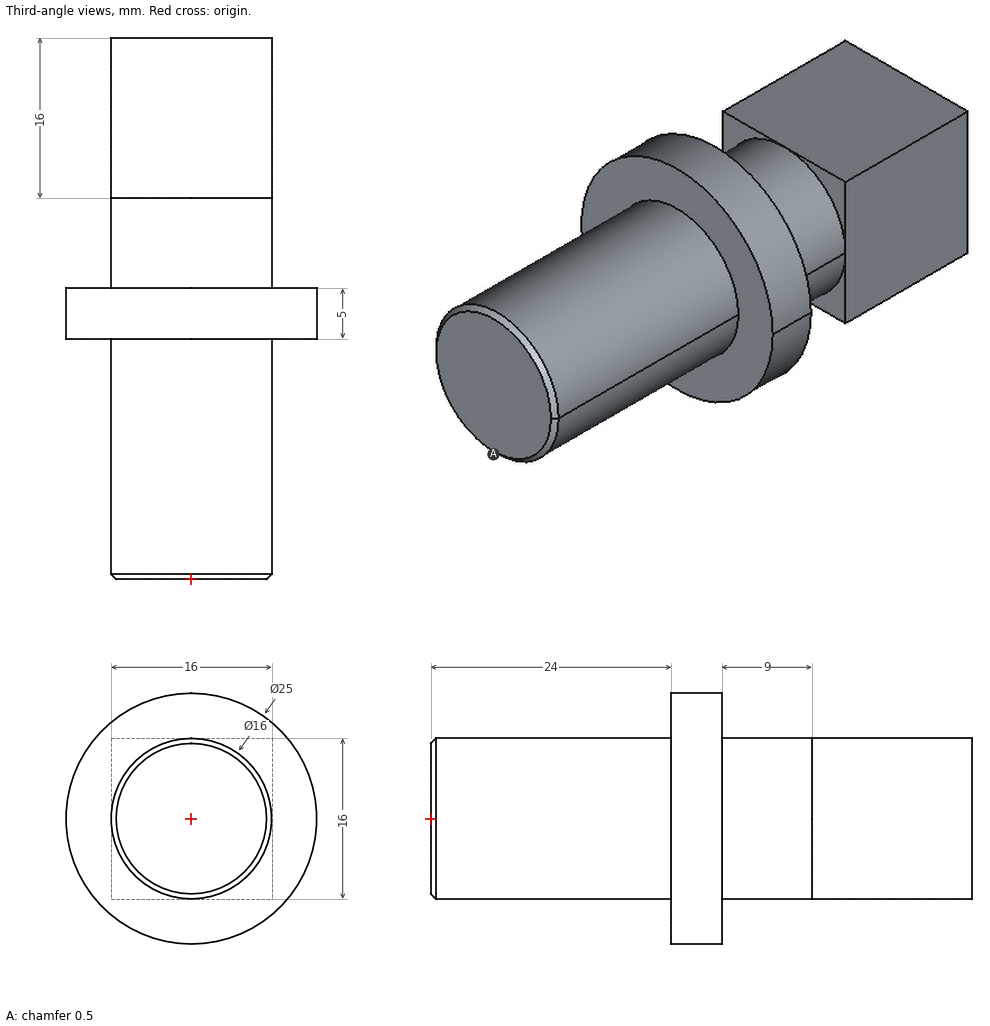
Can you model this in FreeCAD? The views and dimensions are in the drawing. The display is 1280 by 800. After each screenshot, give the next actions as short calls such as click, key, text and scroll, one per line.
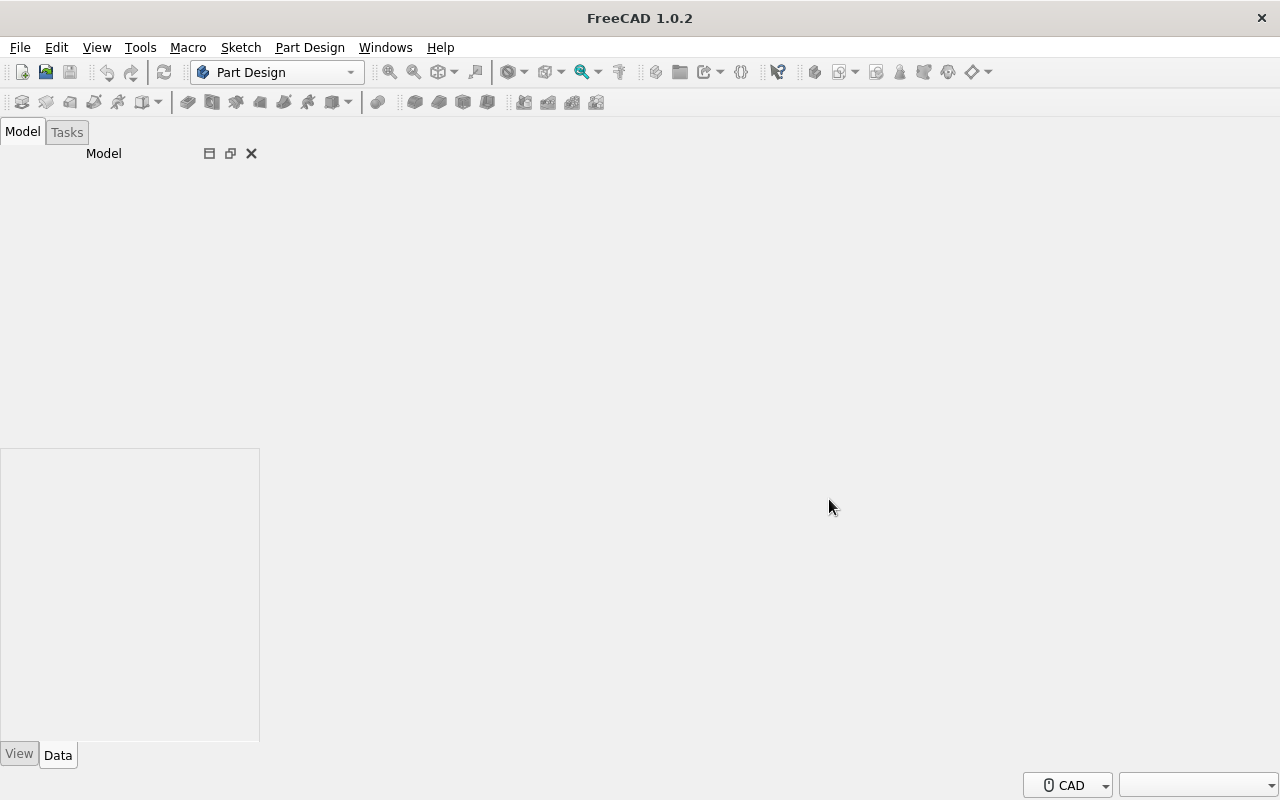
click(22, 72)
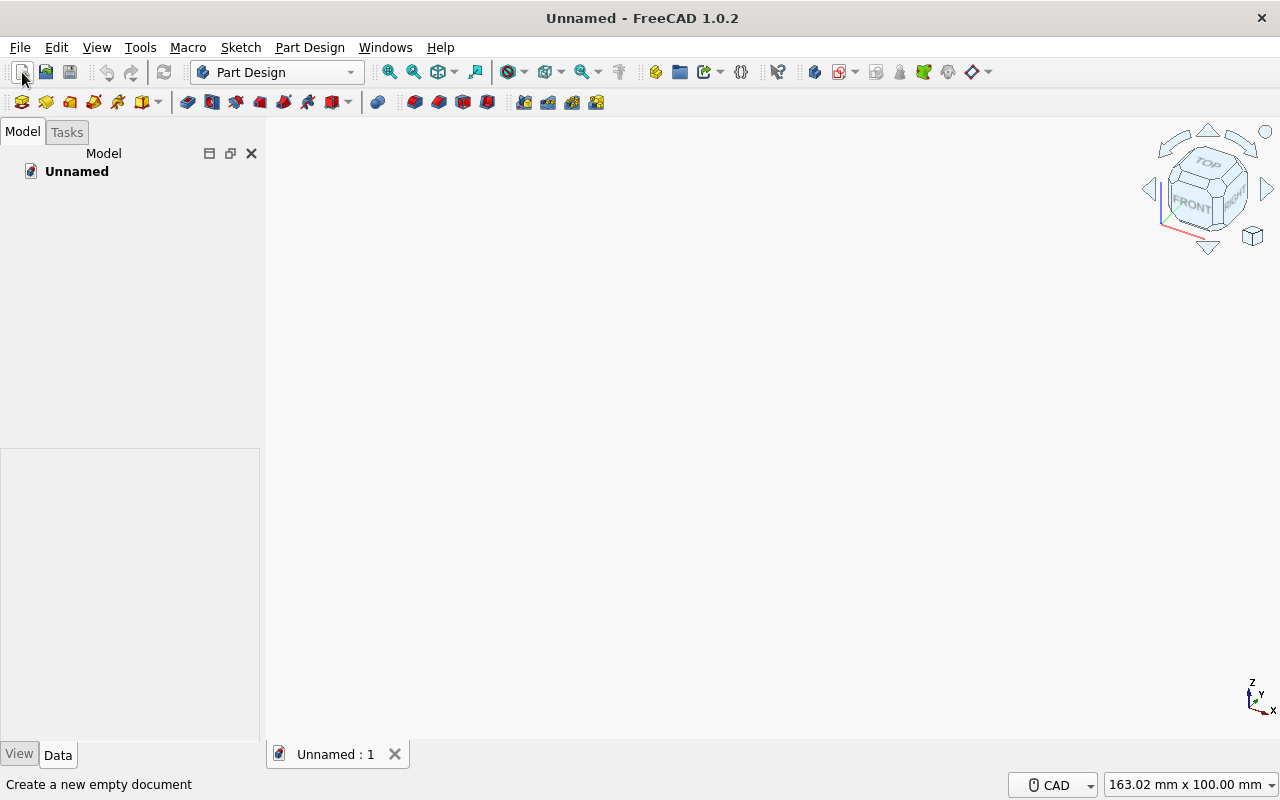
click(840, 72)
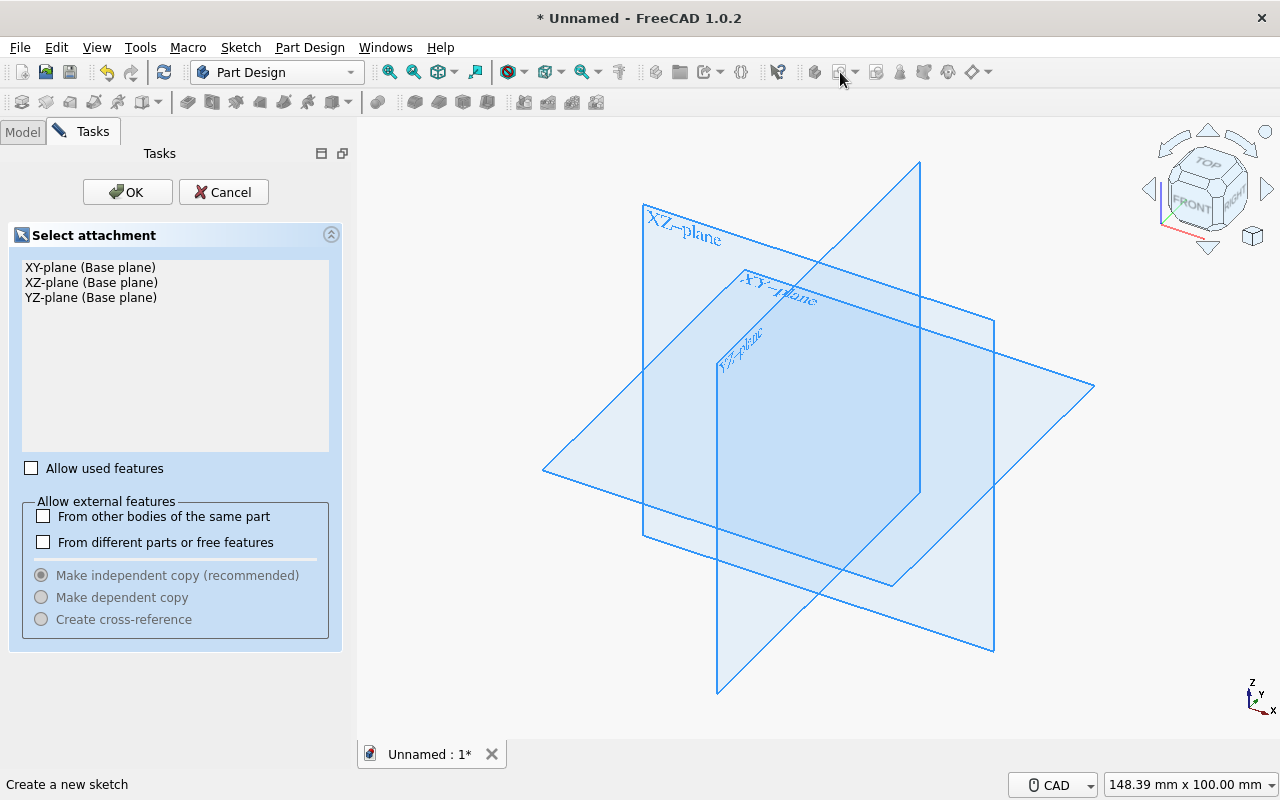
click(82, 282)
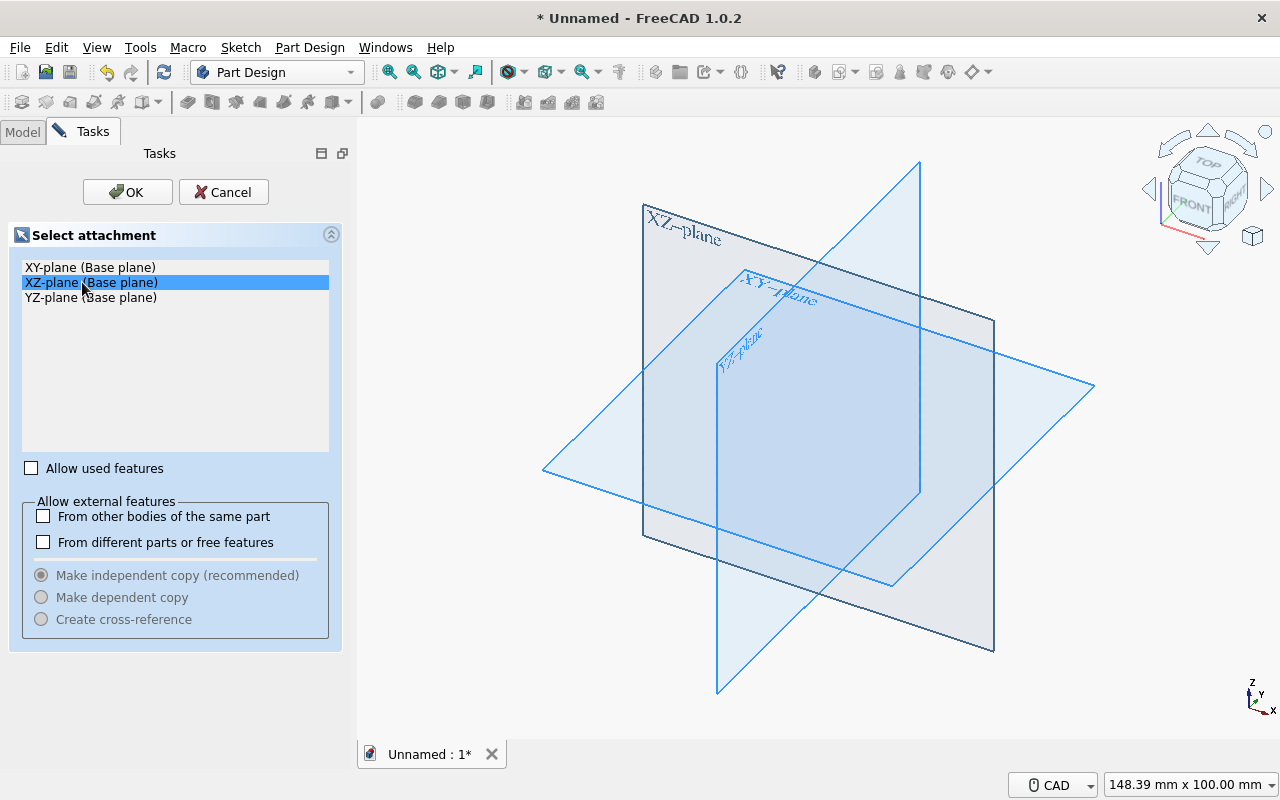
click(128, 192)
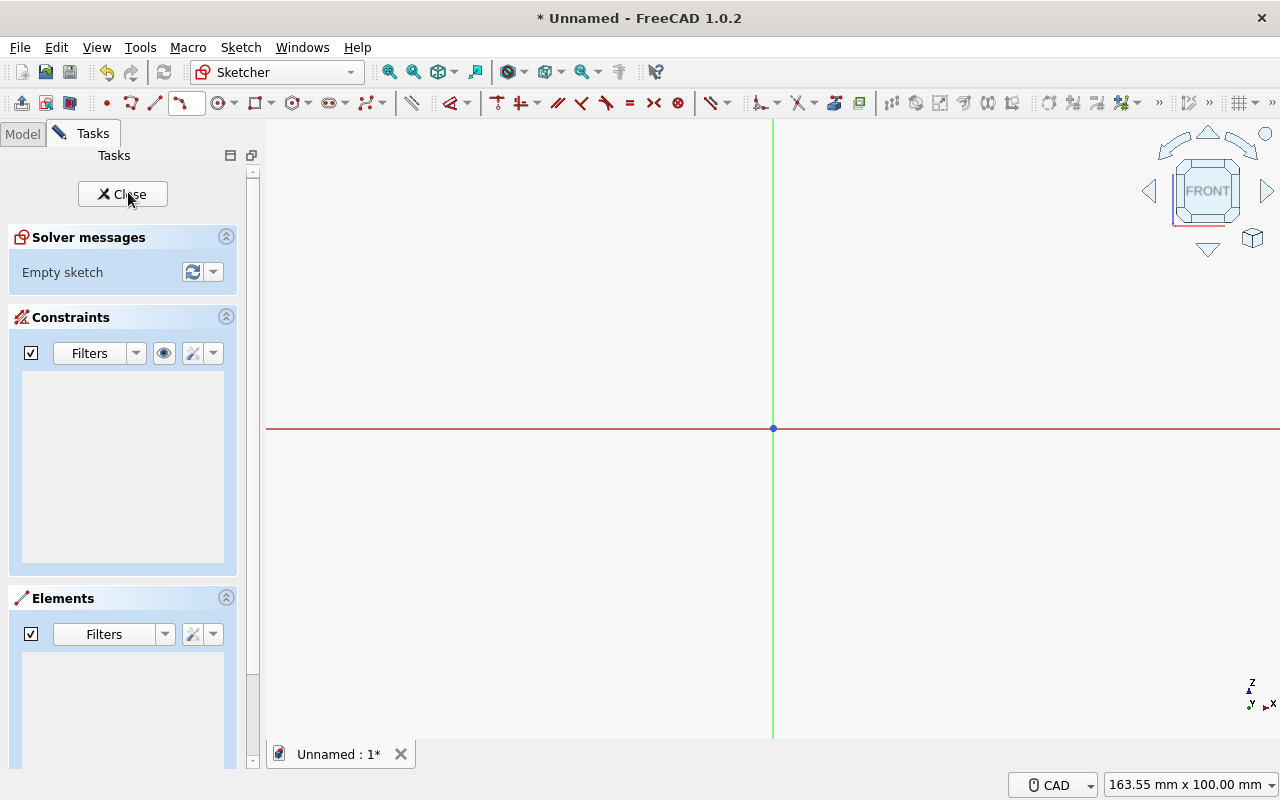
scroll(795, 429, up, 7)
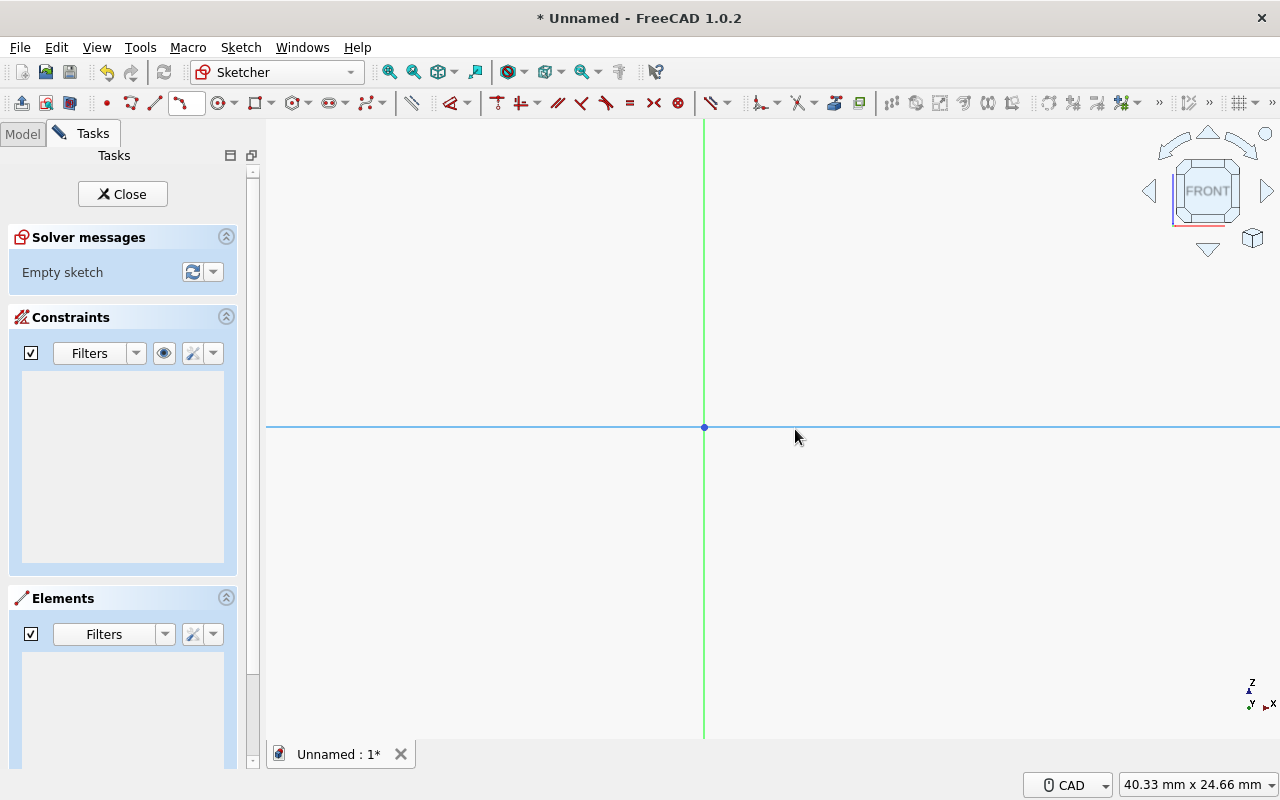
click(218, 104)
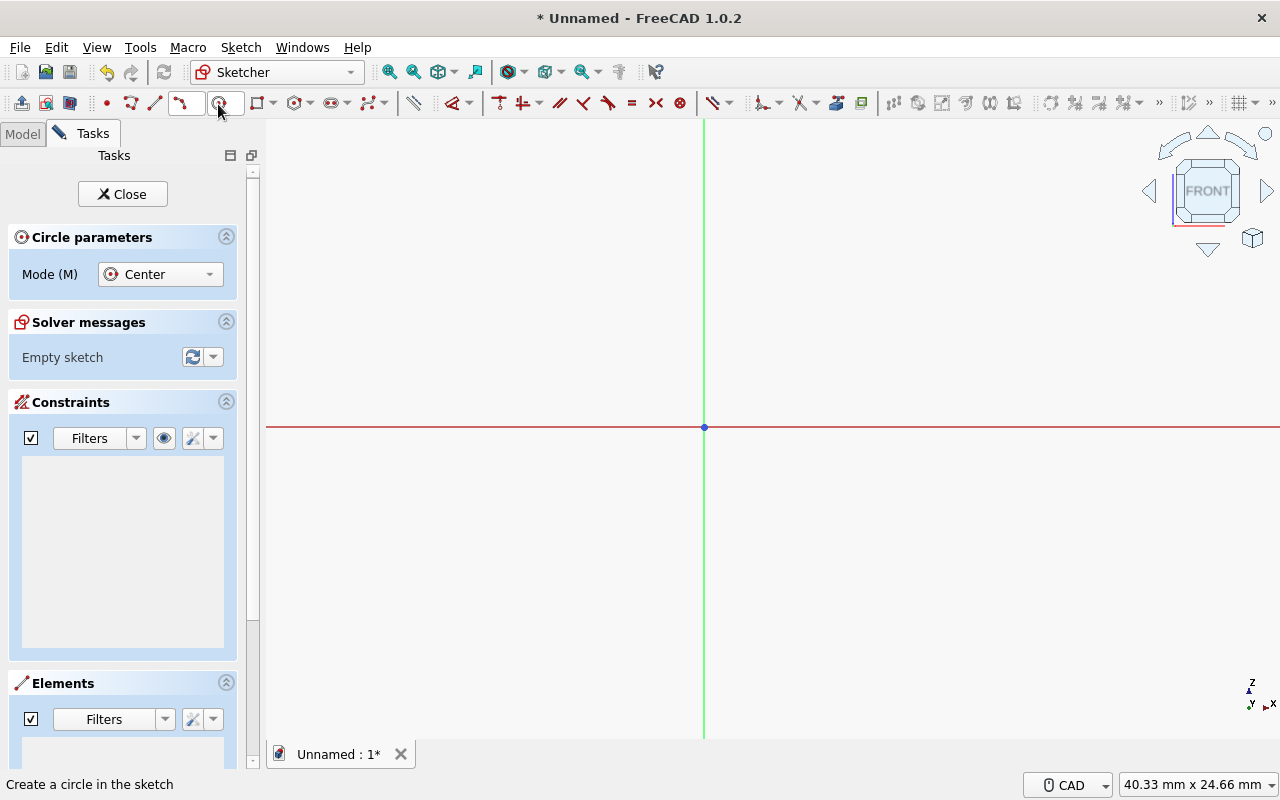
click(704, 427)
move(846, 285)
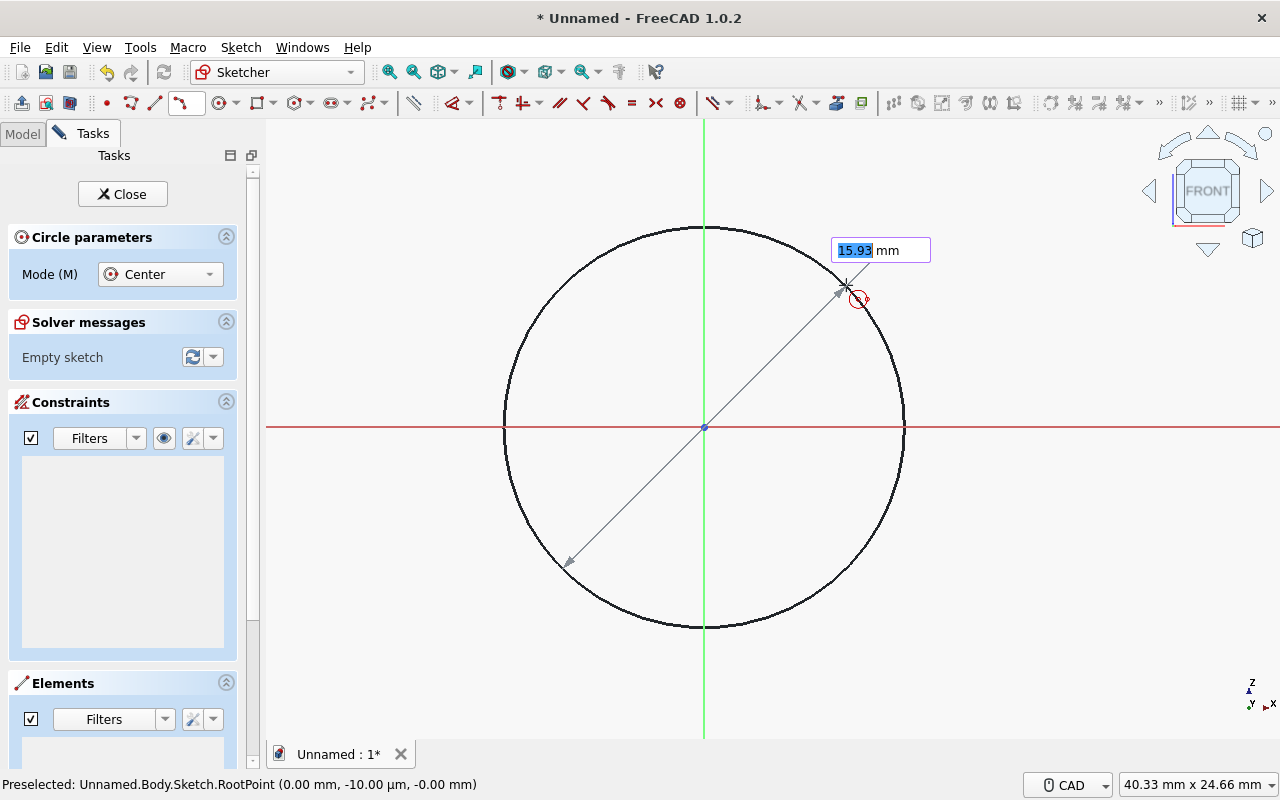
text(16)
key(Return)
key(Escape)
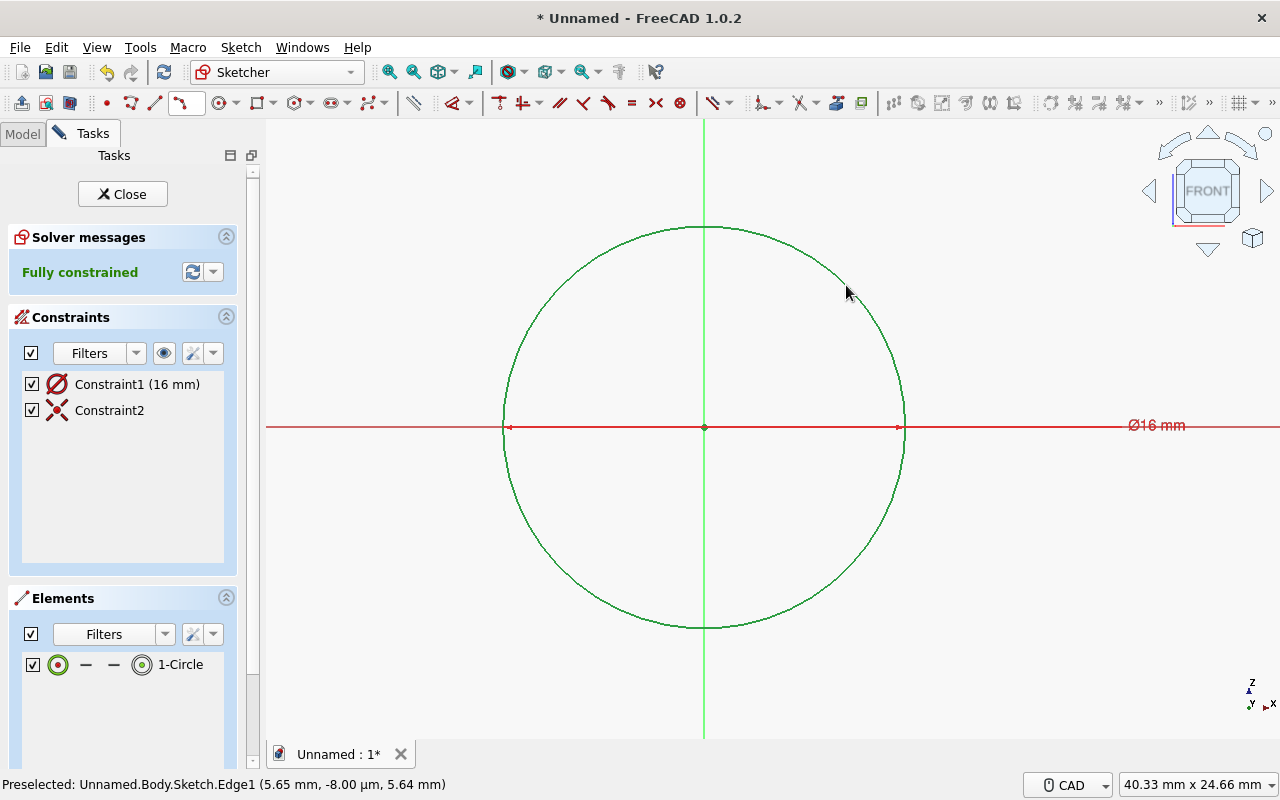
click(123, 194)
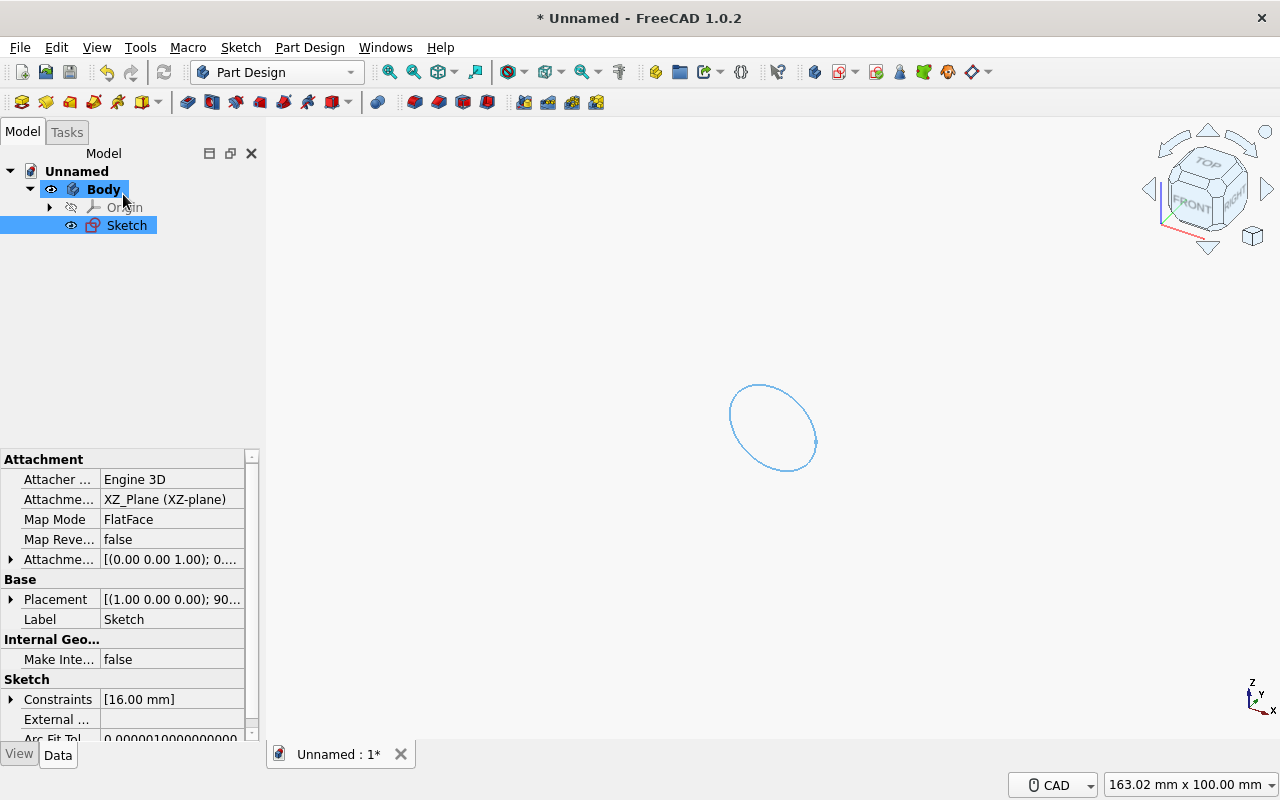
click(22, 102)